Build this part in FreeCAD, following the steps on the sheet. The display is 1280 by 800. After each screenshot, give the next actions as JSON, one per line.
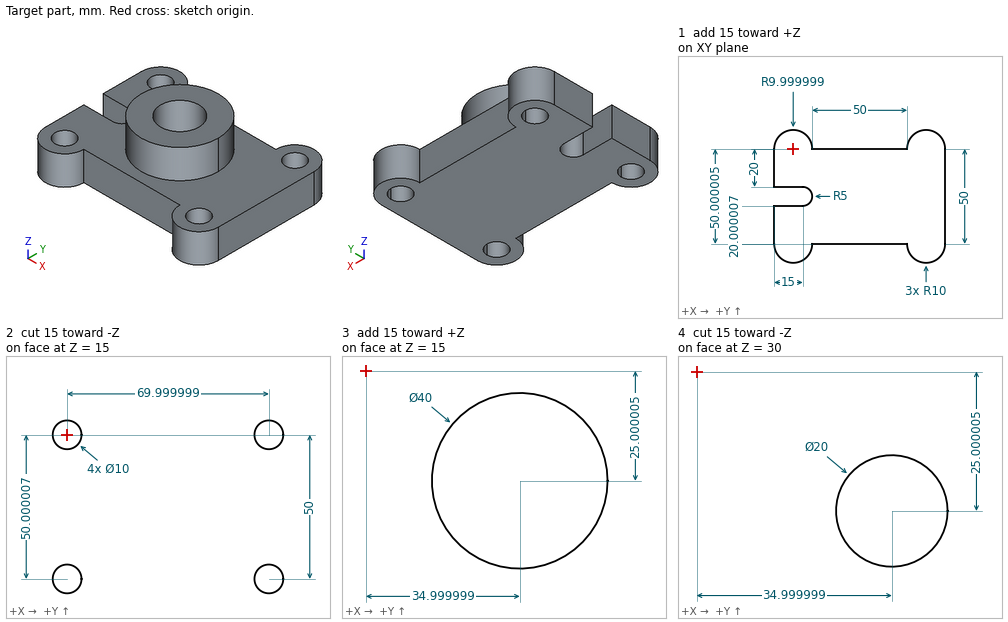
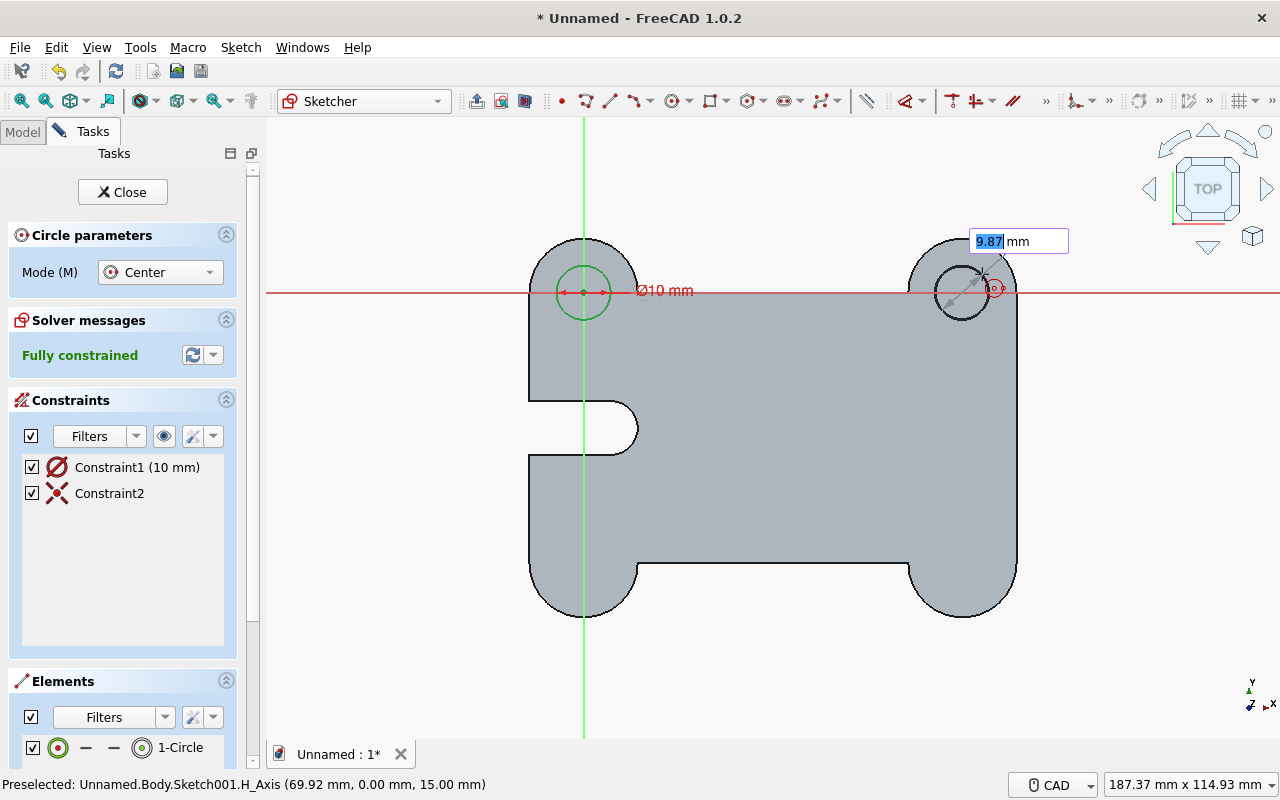
{"action": "type", "text": "10"}
{"action": "key", "text": "Return"}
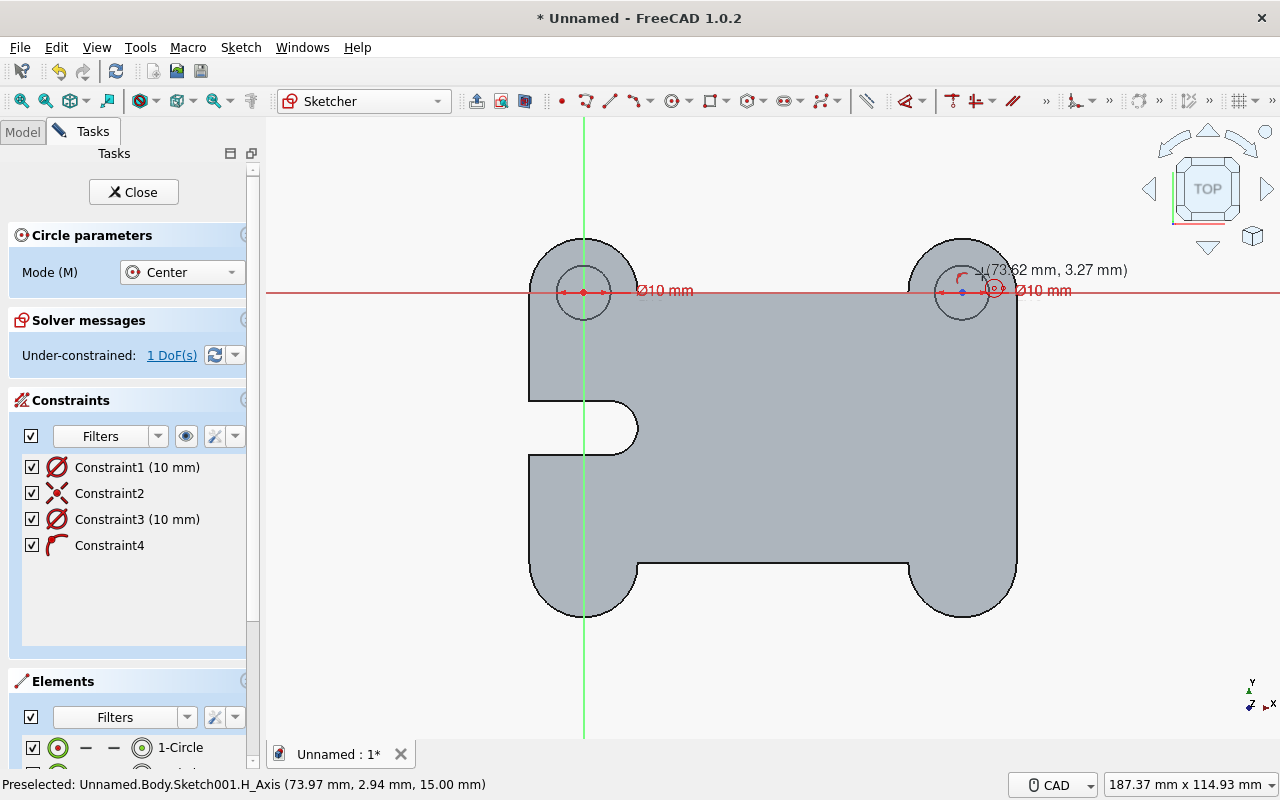
{"action": "left_click", "coordinate": [962, 563]}
{"action": "mouse_move", "coordinate": [982, 544]}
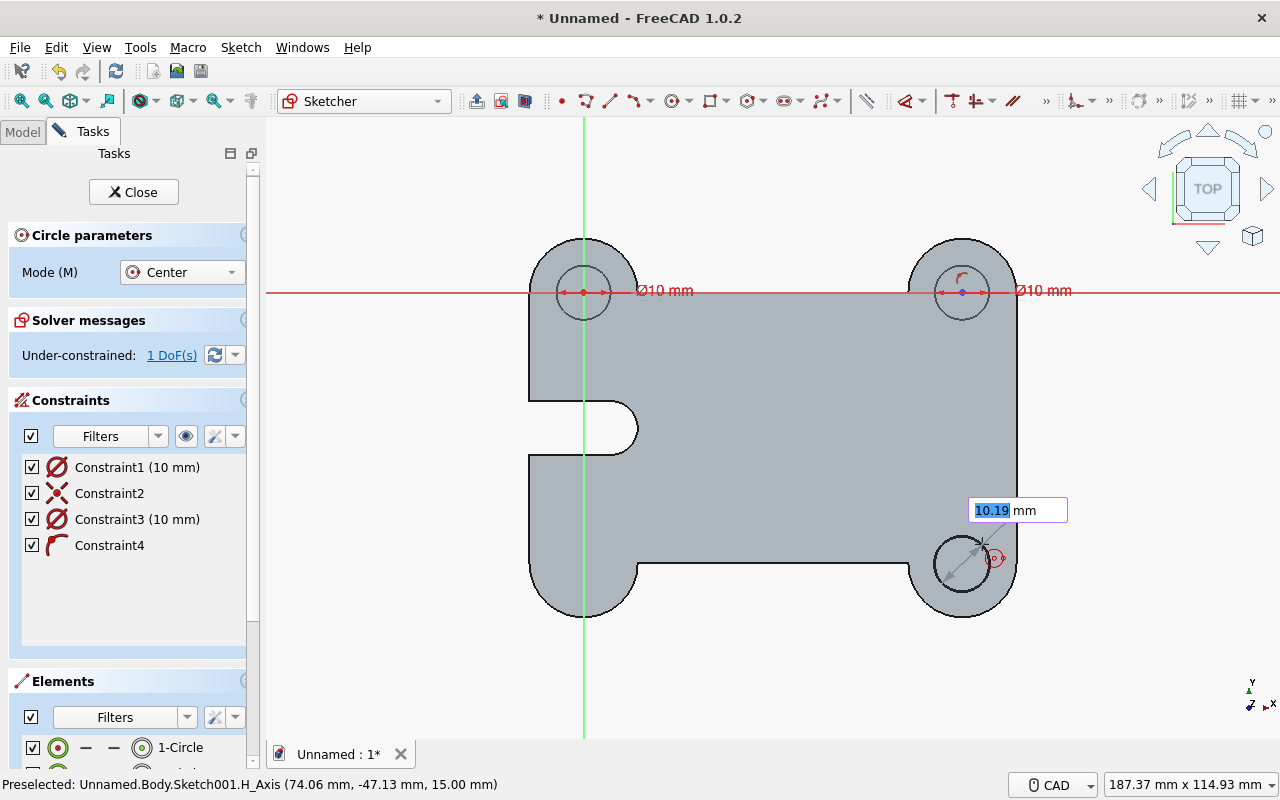
{"action": "type", "text": "10"}
{"action": "key", "text": "Return"}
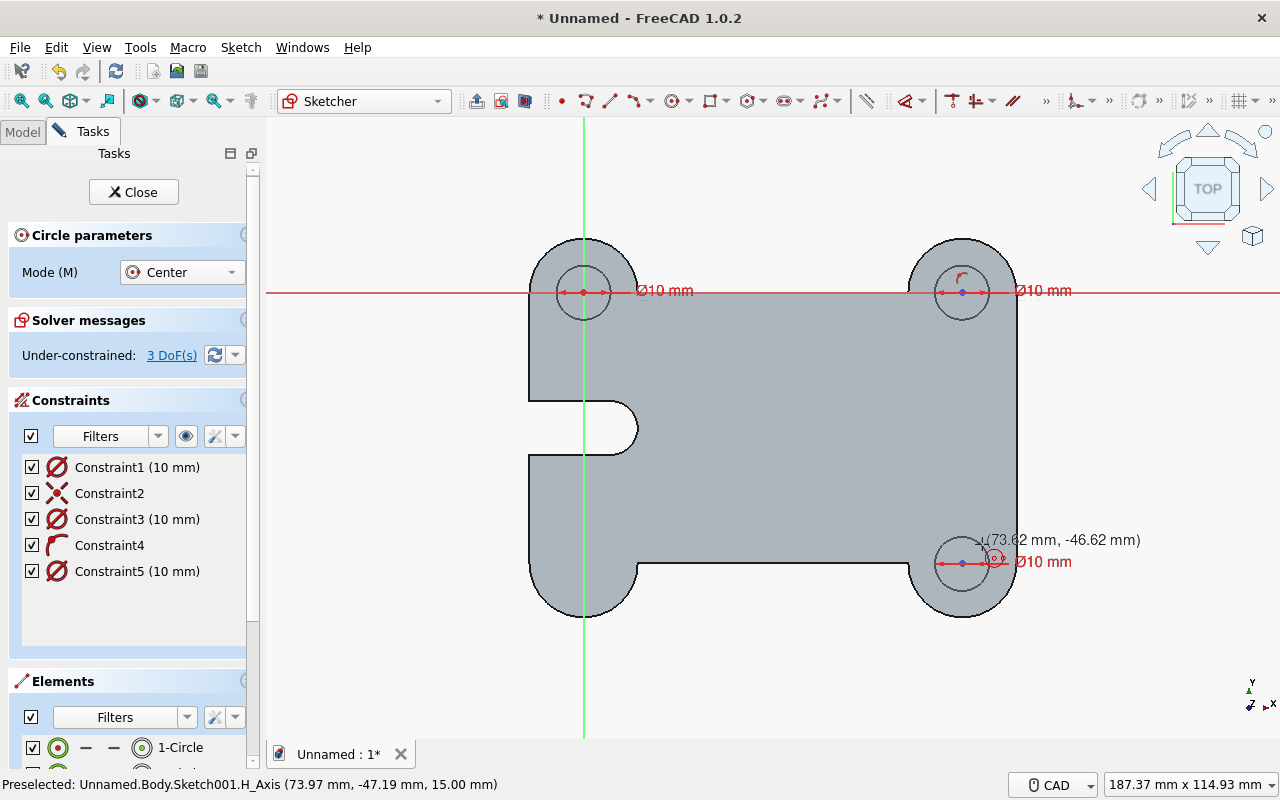
{"action": "left_click", "coordinate": [584, 563]}
{"action": "mouse_move", "coordinate": [603, 544]}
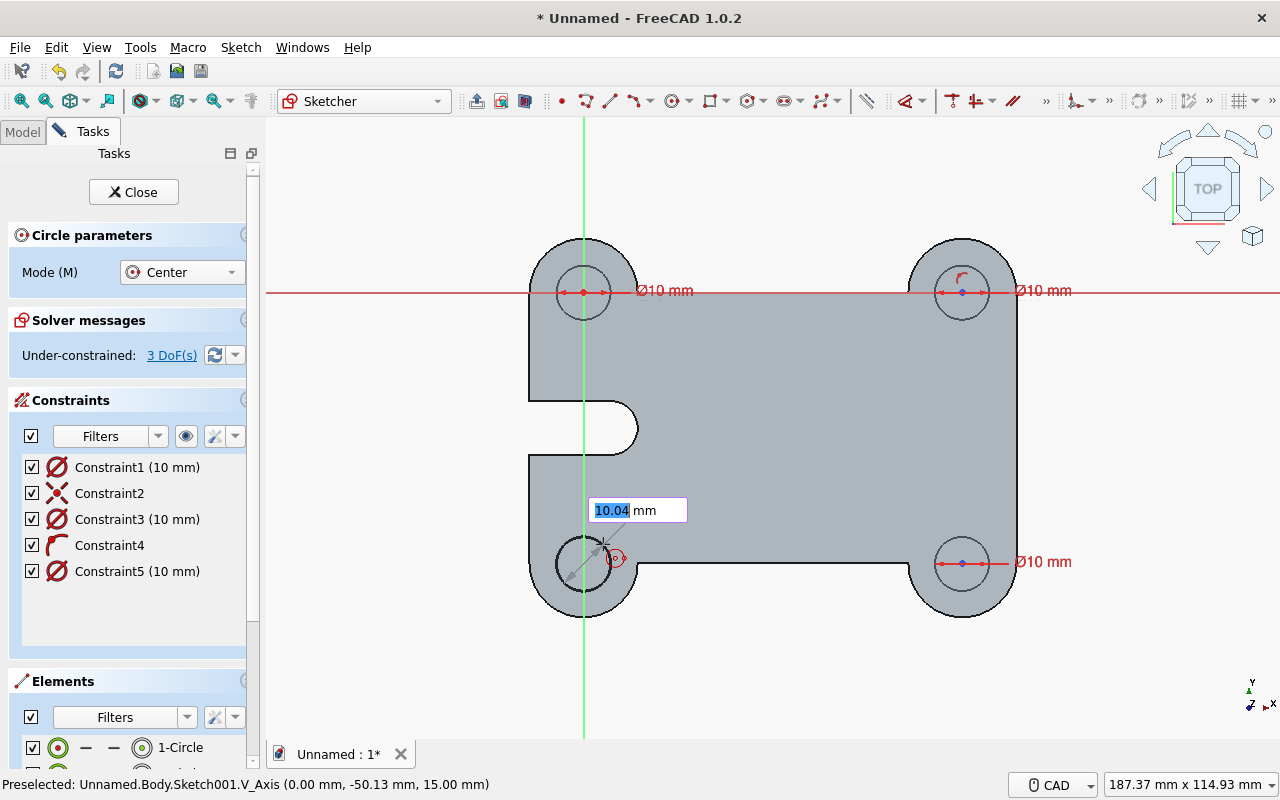
{"action": "type", "text": "10"}
{"action": "key", "text": "Return"}
{"action": "key", "text": "Escape"}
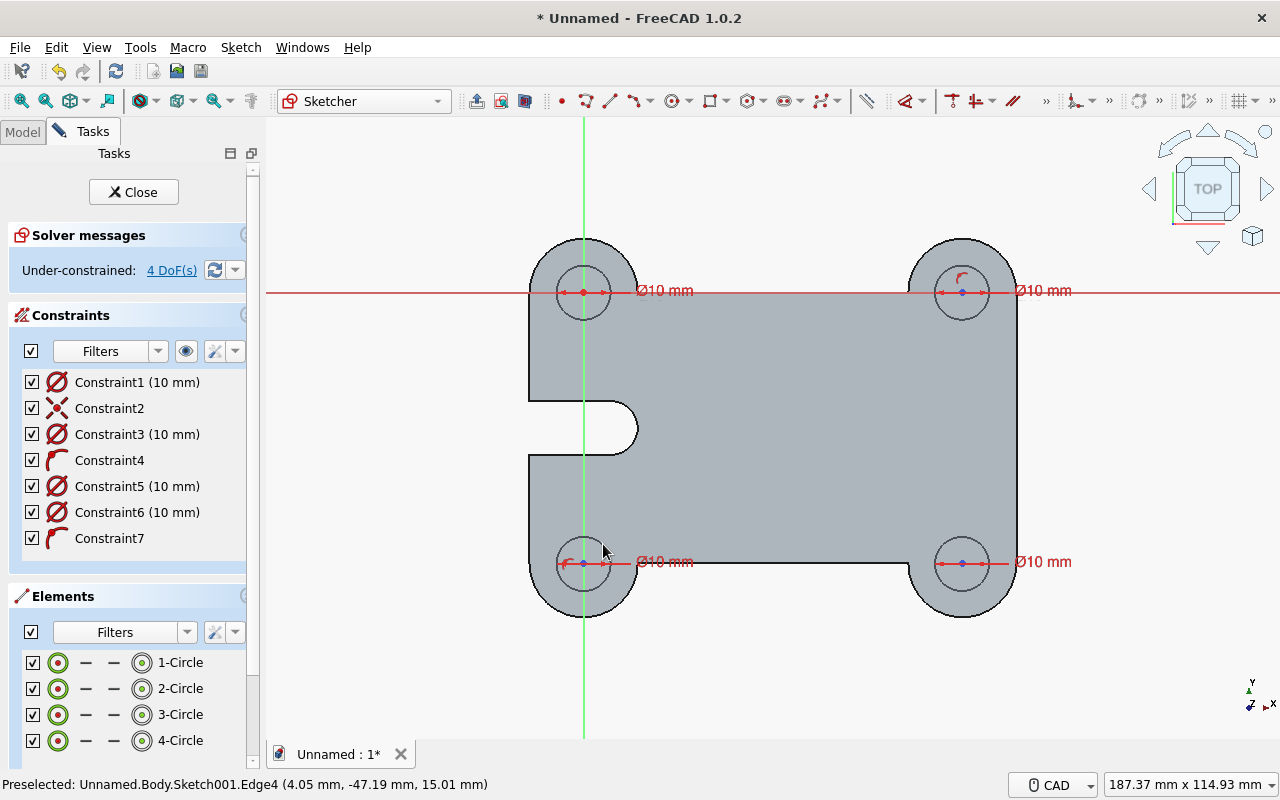
{"action": "left_click", "coordinate": [962, 293]}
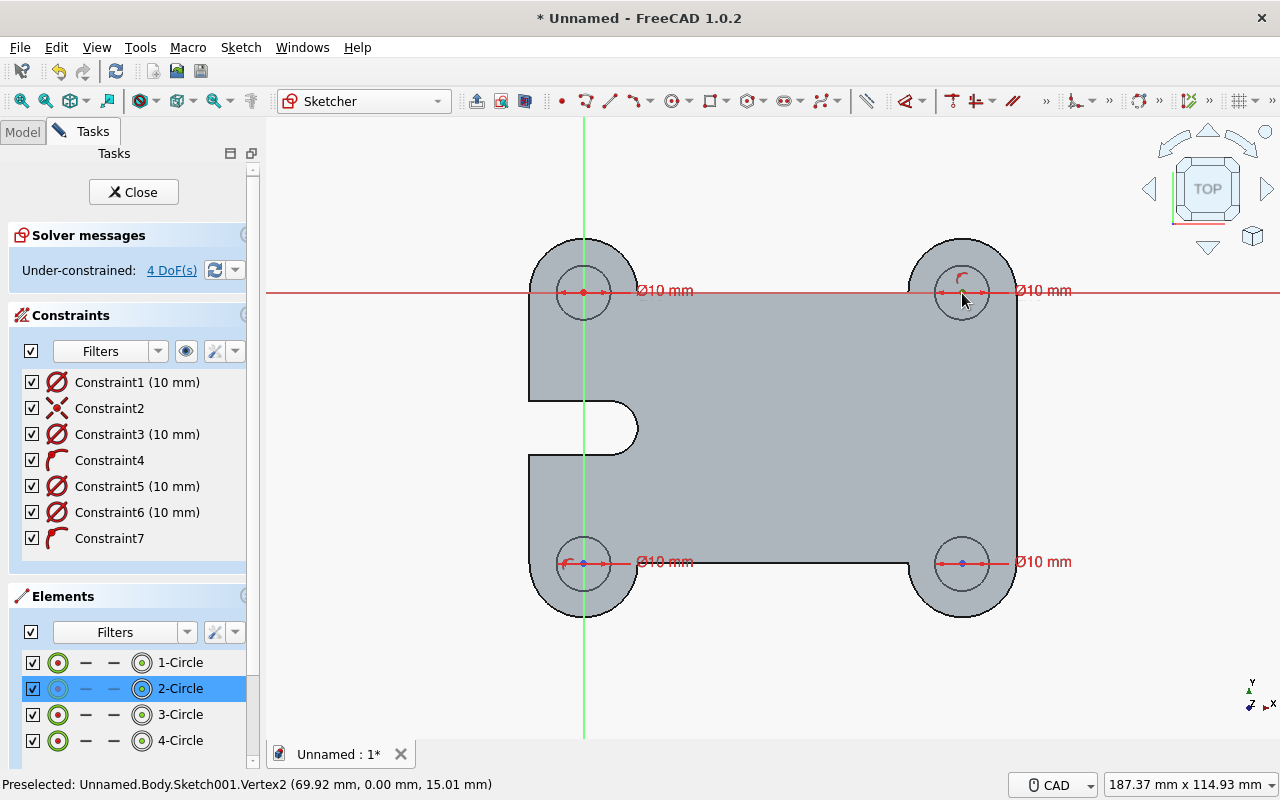
{"action": "left_click", "coordinate": [962, 564]}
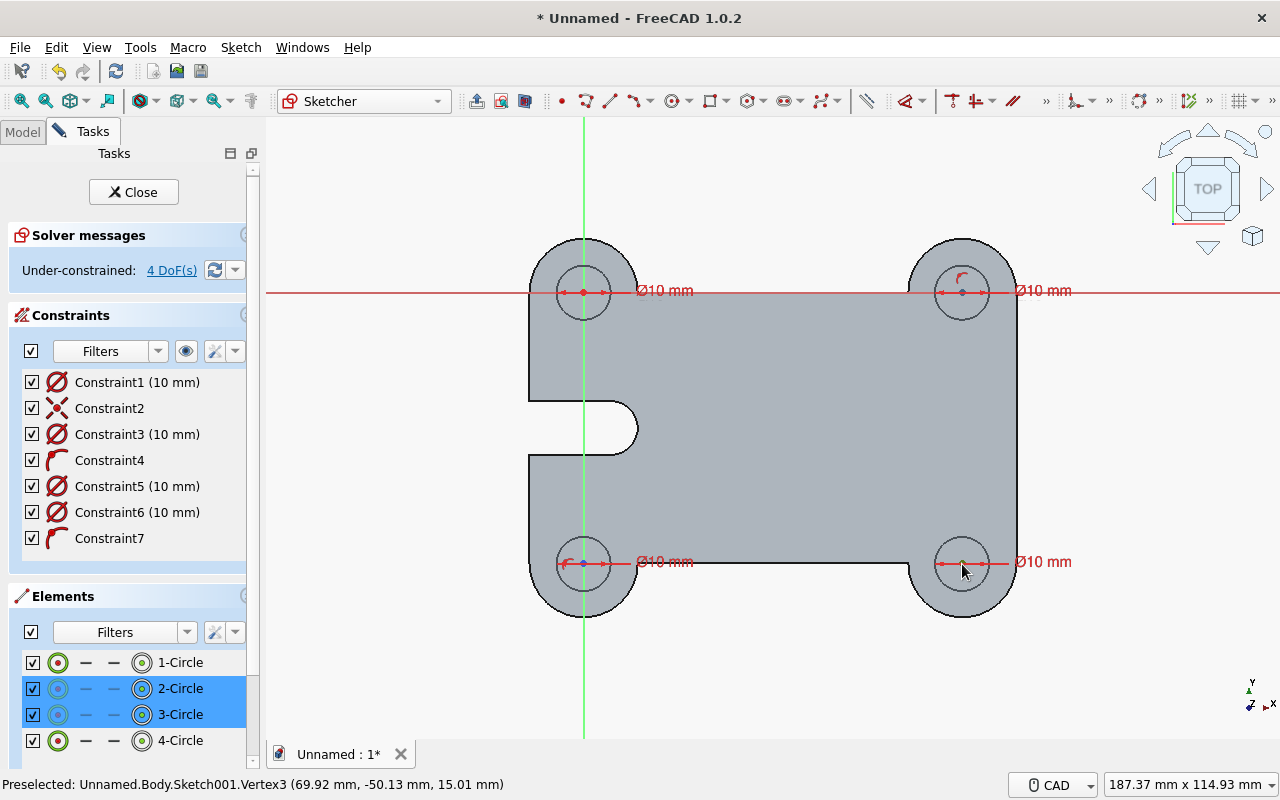
{"action": "key", "text": "v"}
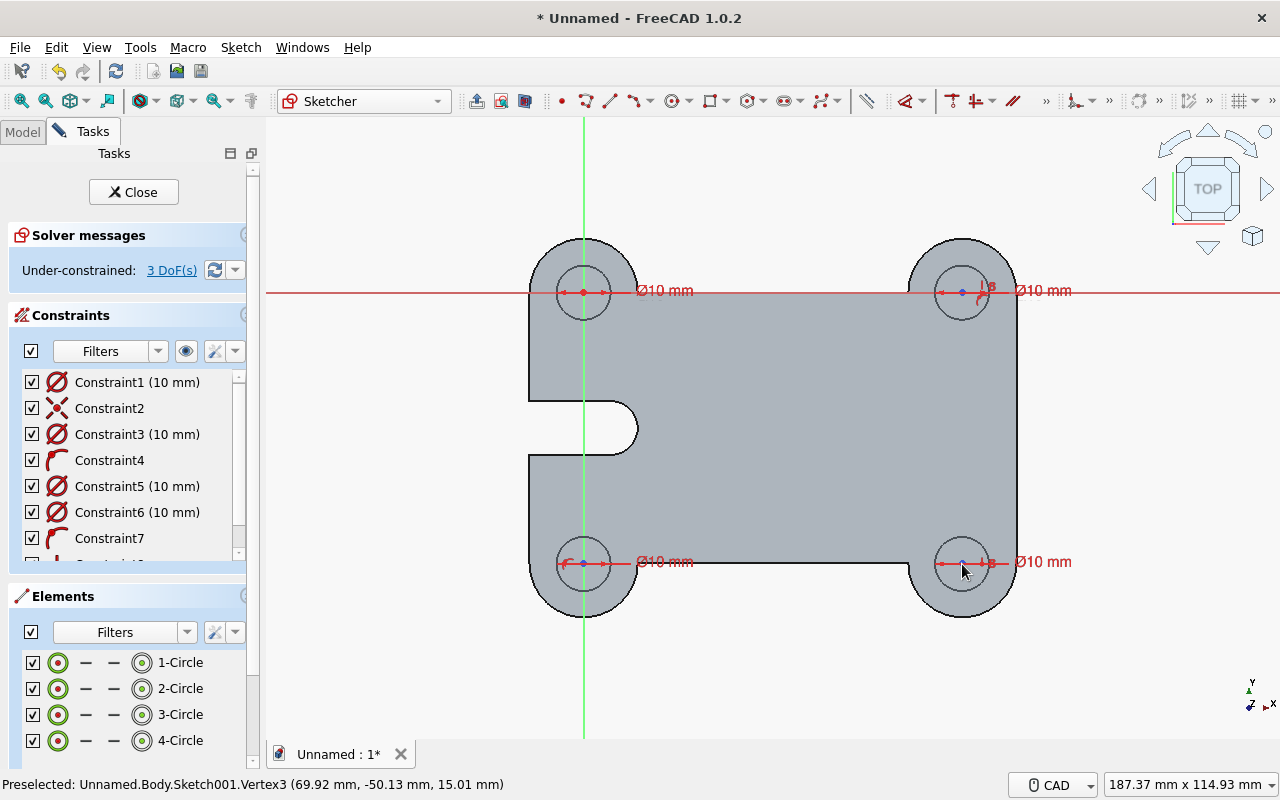
{"action": "left_click", "coordinate": [906, 102]}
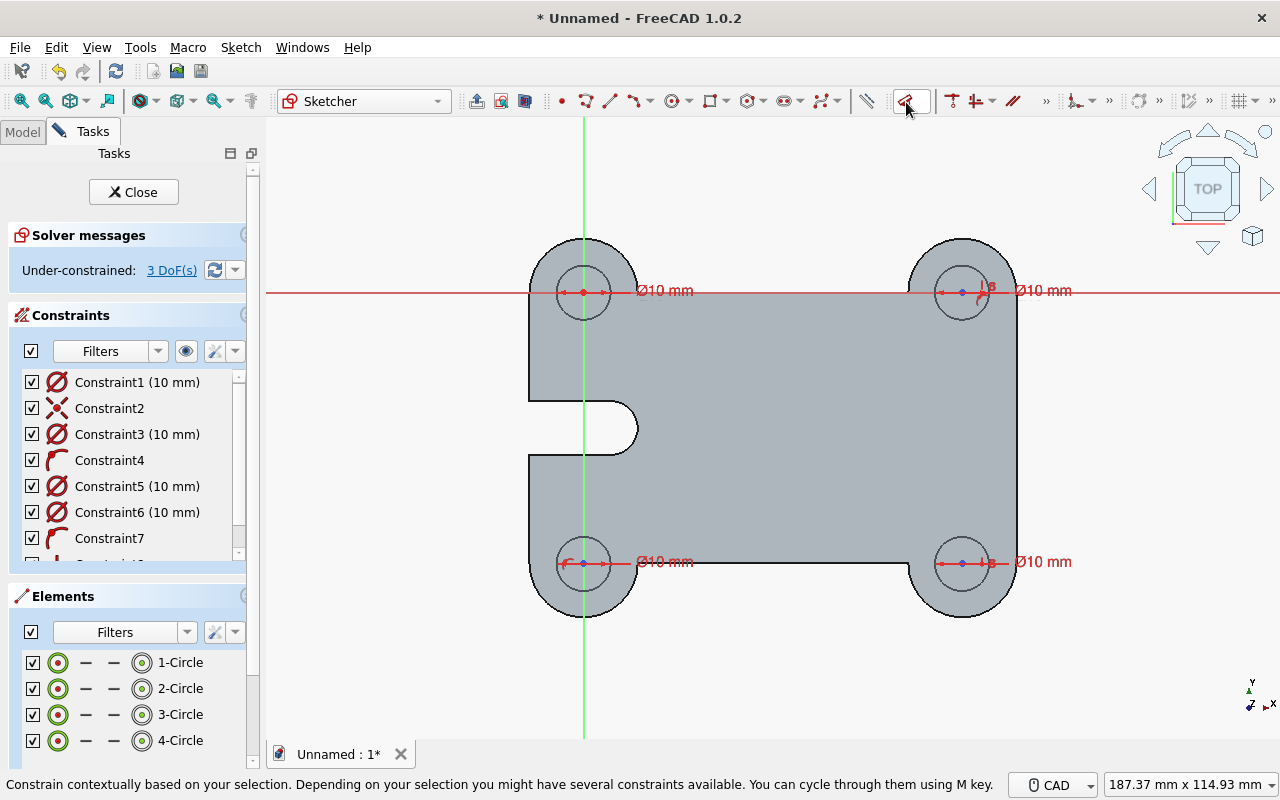
{"action": "left_click", "coordinate": [962, 564]}
{"action": "left_click", "coordinate": [550, 428]}